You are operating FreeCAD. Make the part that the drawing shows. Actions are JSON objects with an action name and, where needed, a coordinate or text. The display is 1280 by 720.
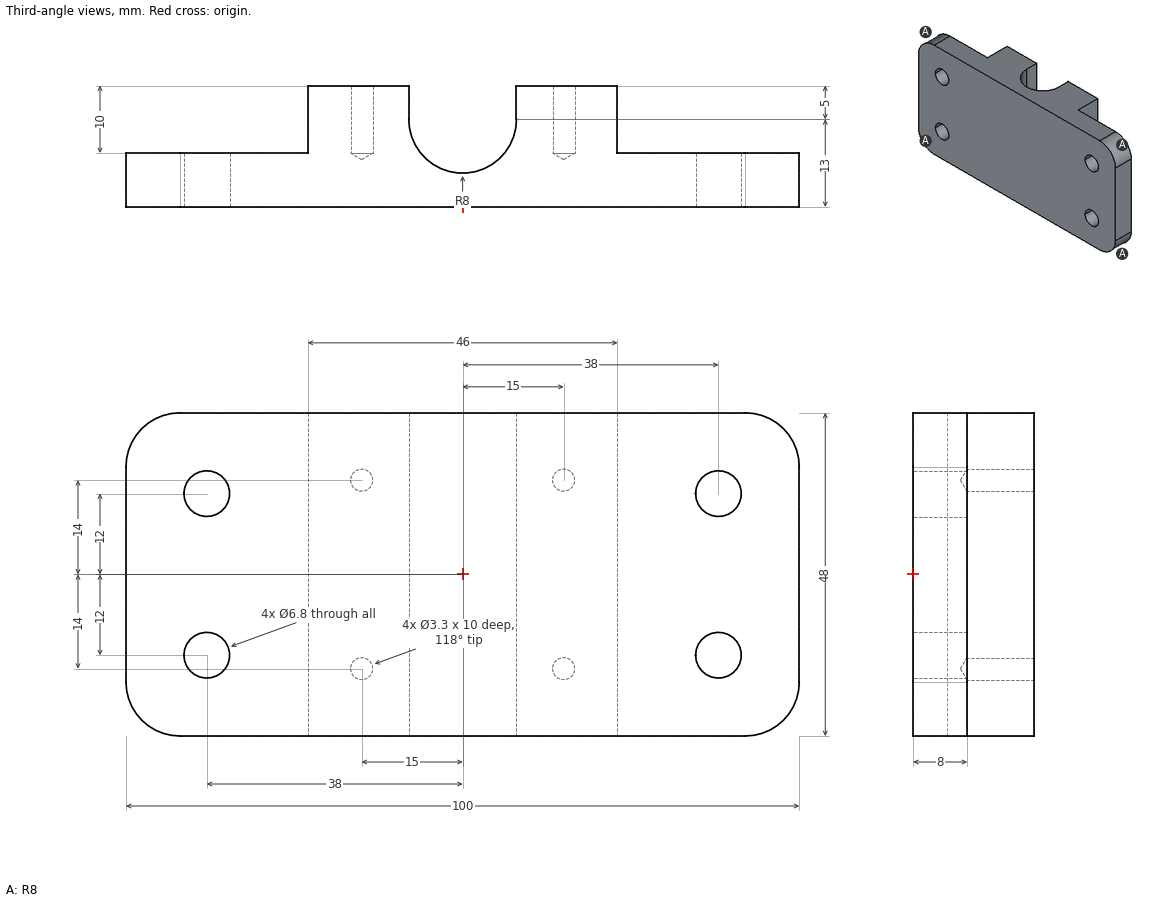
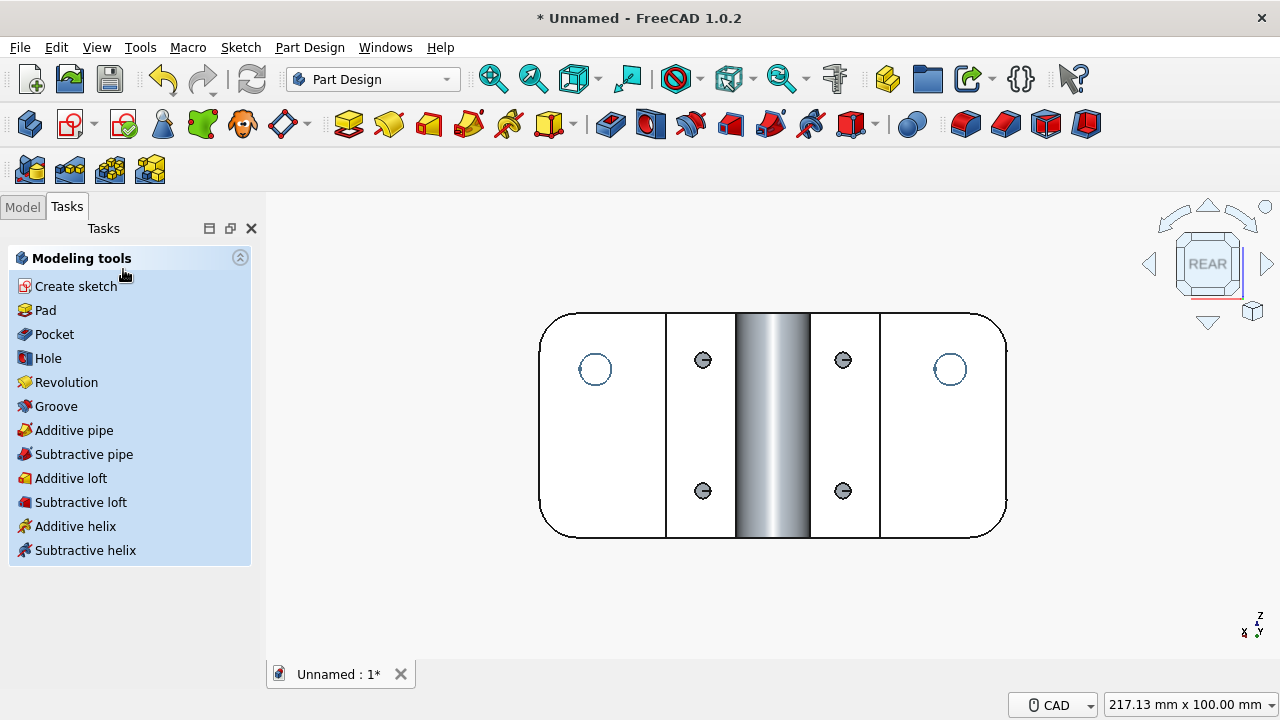
{"action": "left_click", "coordinate": [652, 124]}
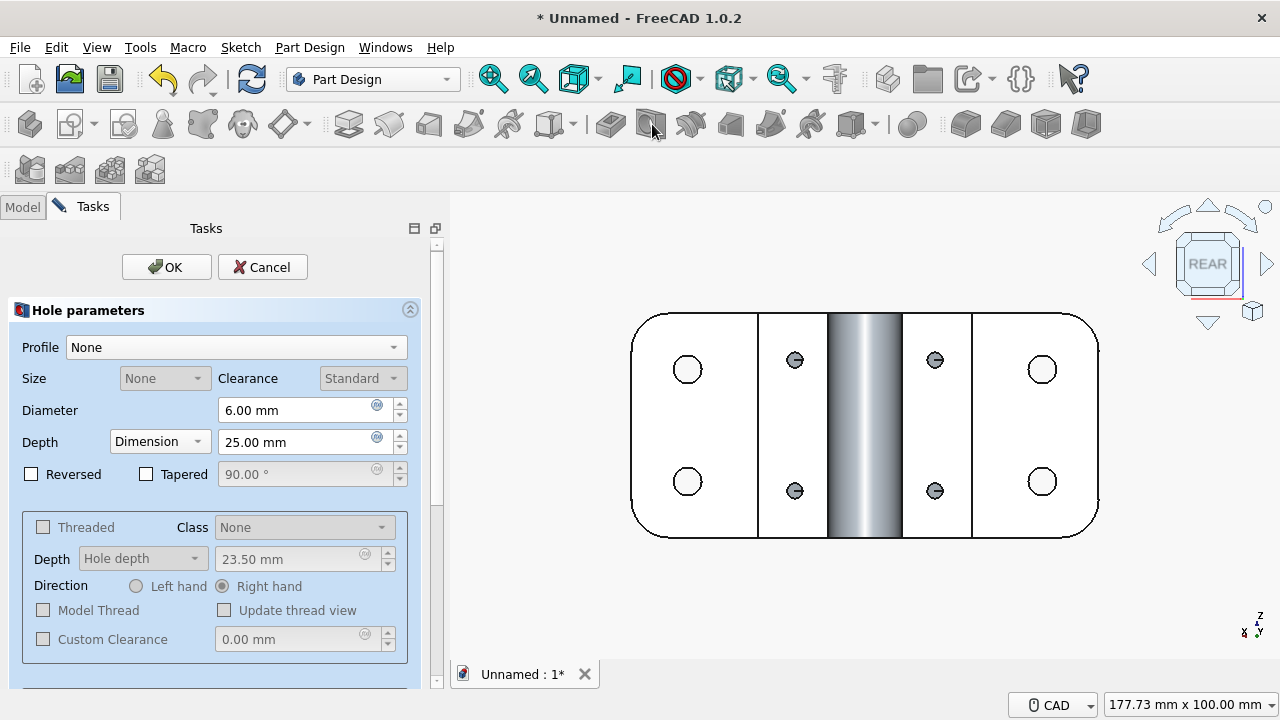
{"action": "triple_click", "coordinate": [305, 410]}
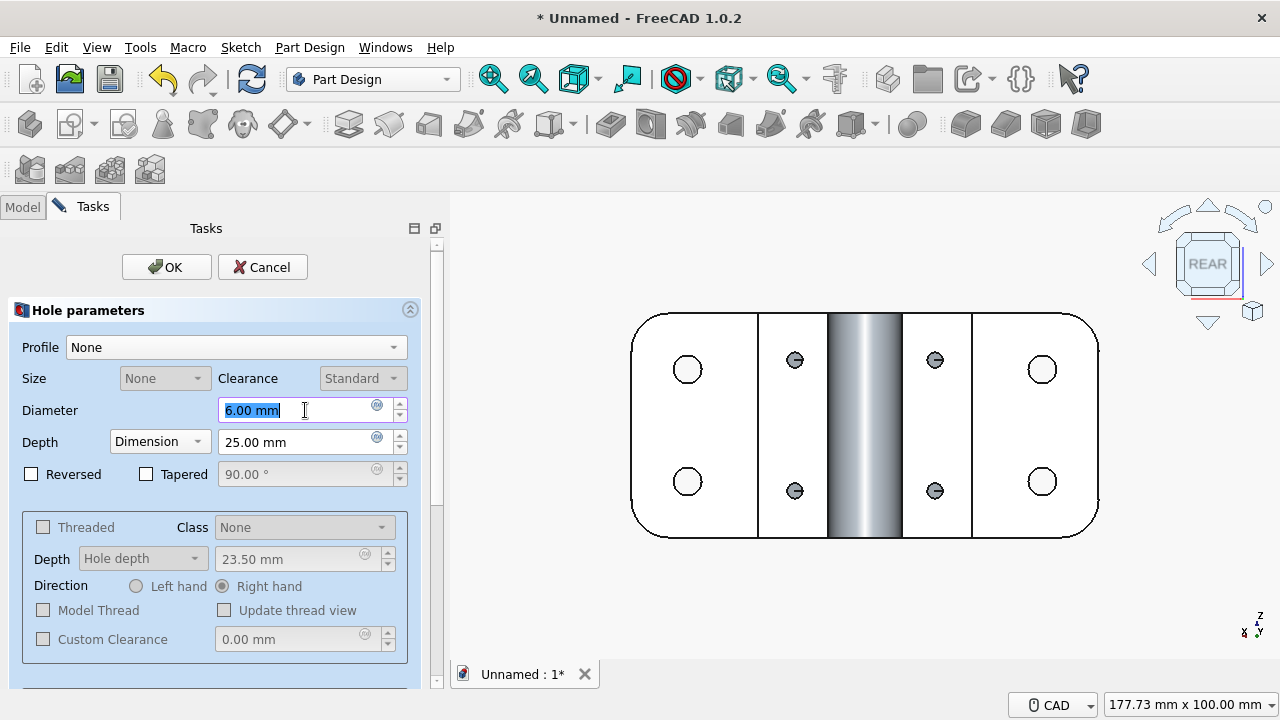
{"action": "type", "text": "6.8"}
{"action": "key", "text": "Tab"}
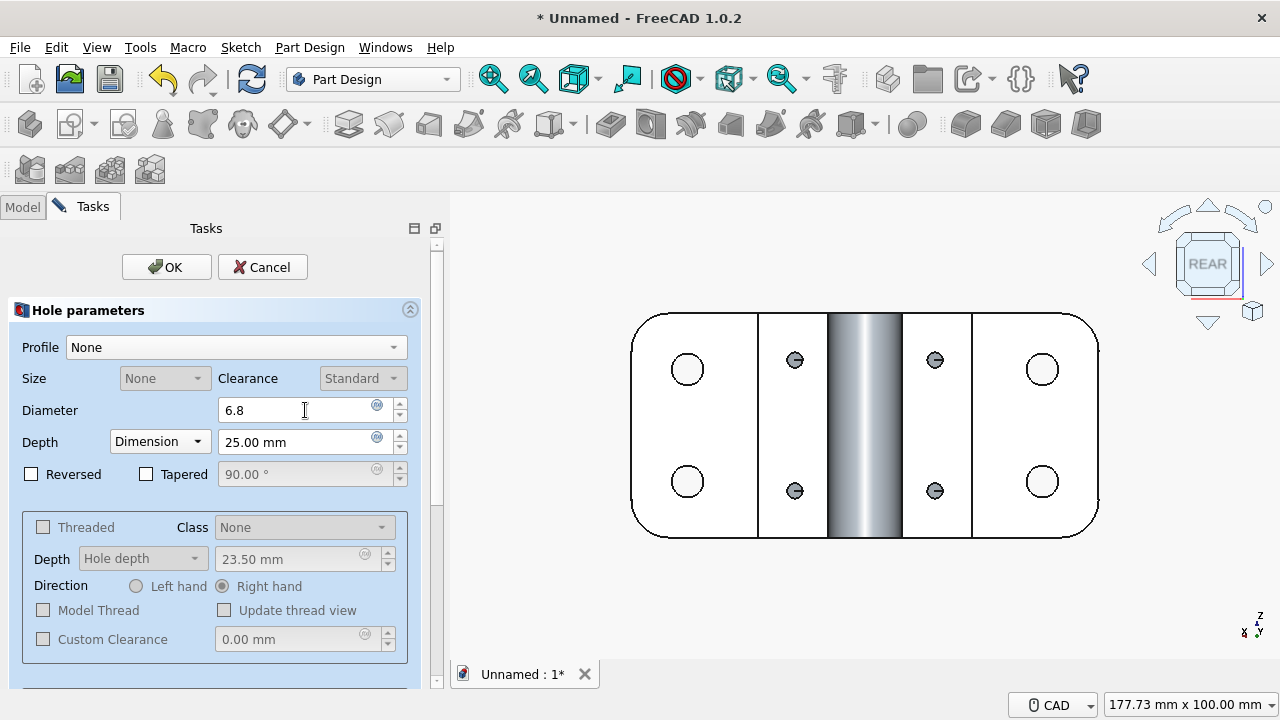
{"action": "left_click", "coordinate": [161, 442]}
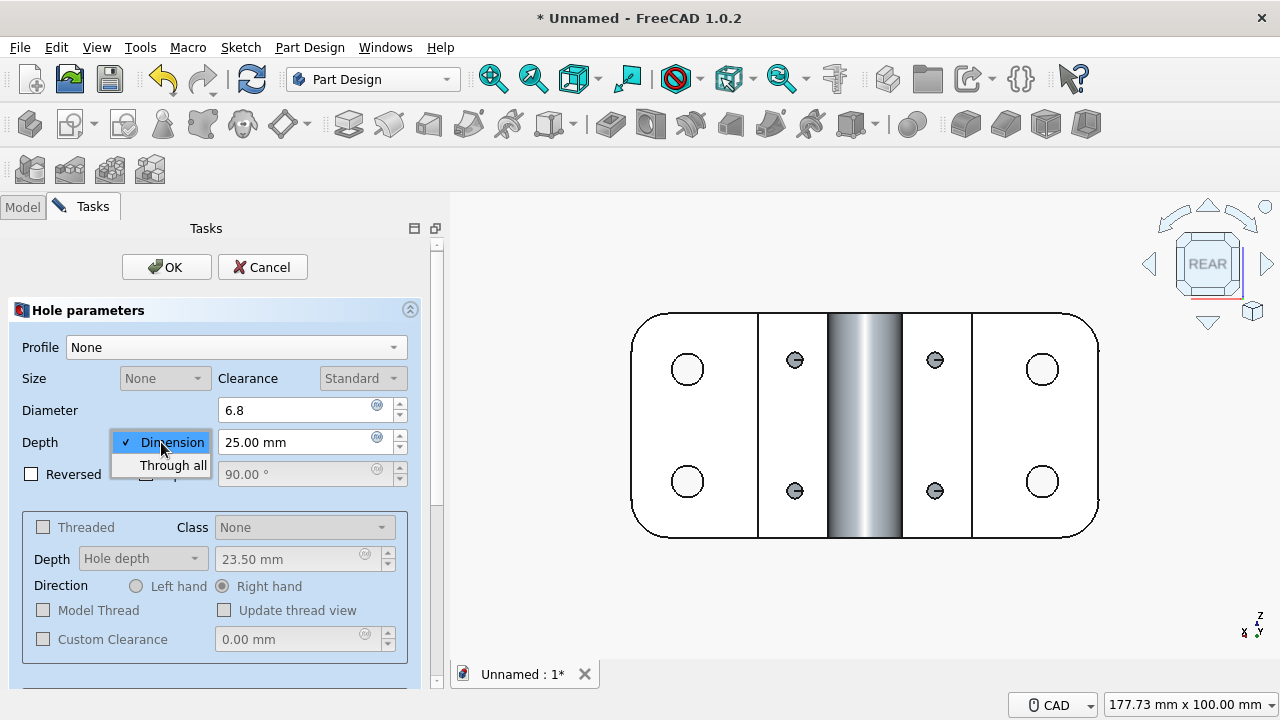
{"action": "left_click", "coordinate": [160, 466]}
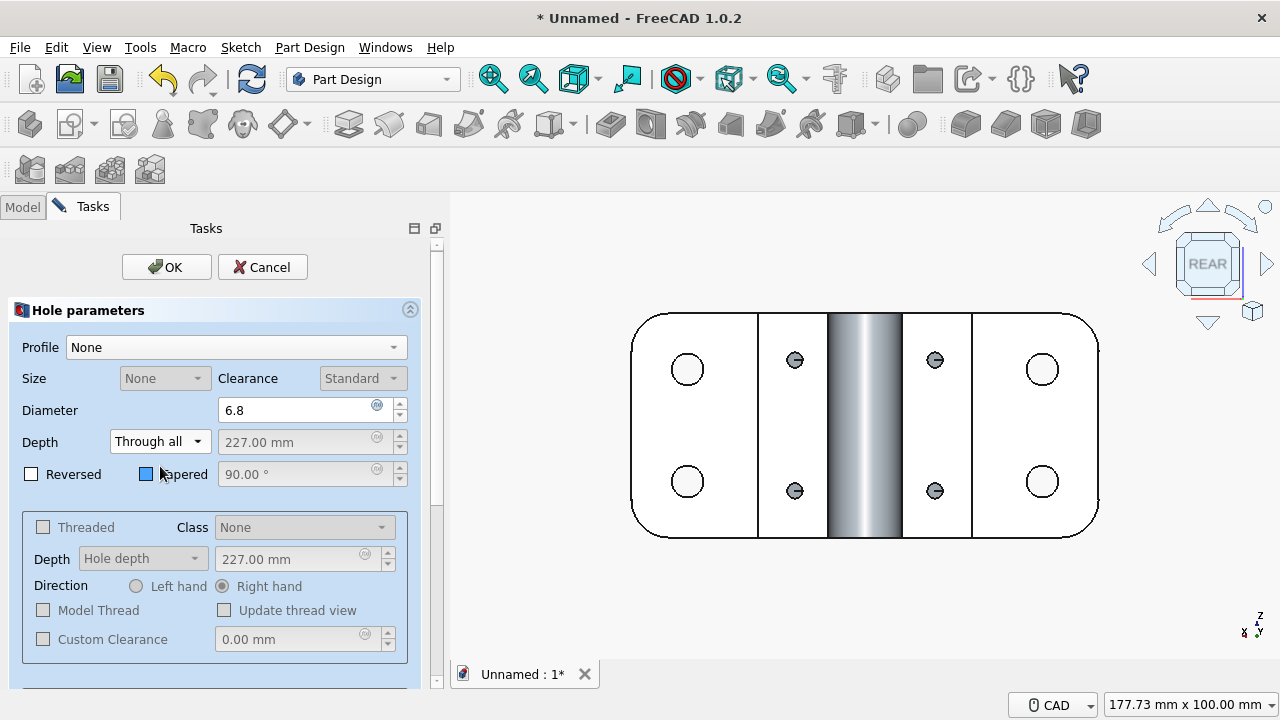
{"action": "left_click", "coordinate": [167, 267]}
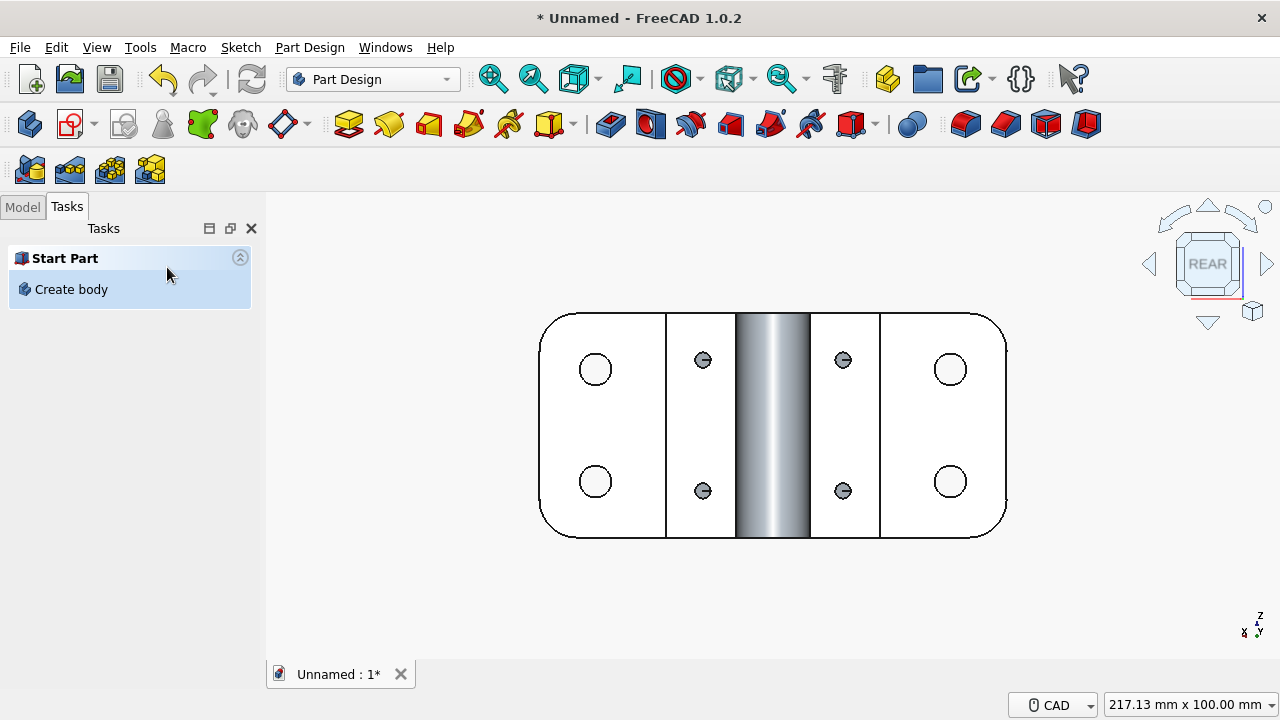
{"action": "key", "text": "0"}